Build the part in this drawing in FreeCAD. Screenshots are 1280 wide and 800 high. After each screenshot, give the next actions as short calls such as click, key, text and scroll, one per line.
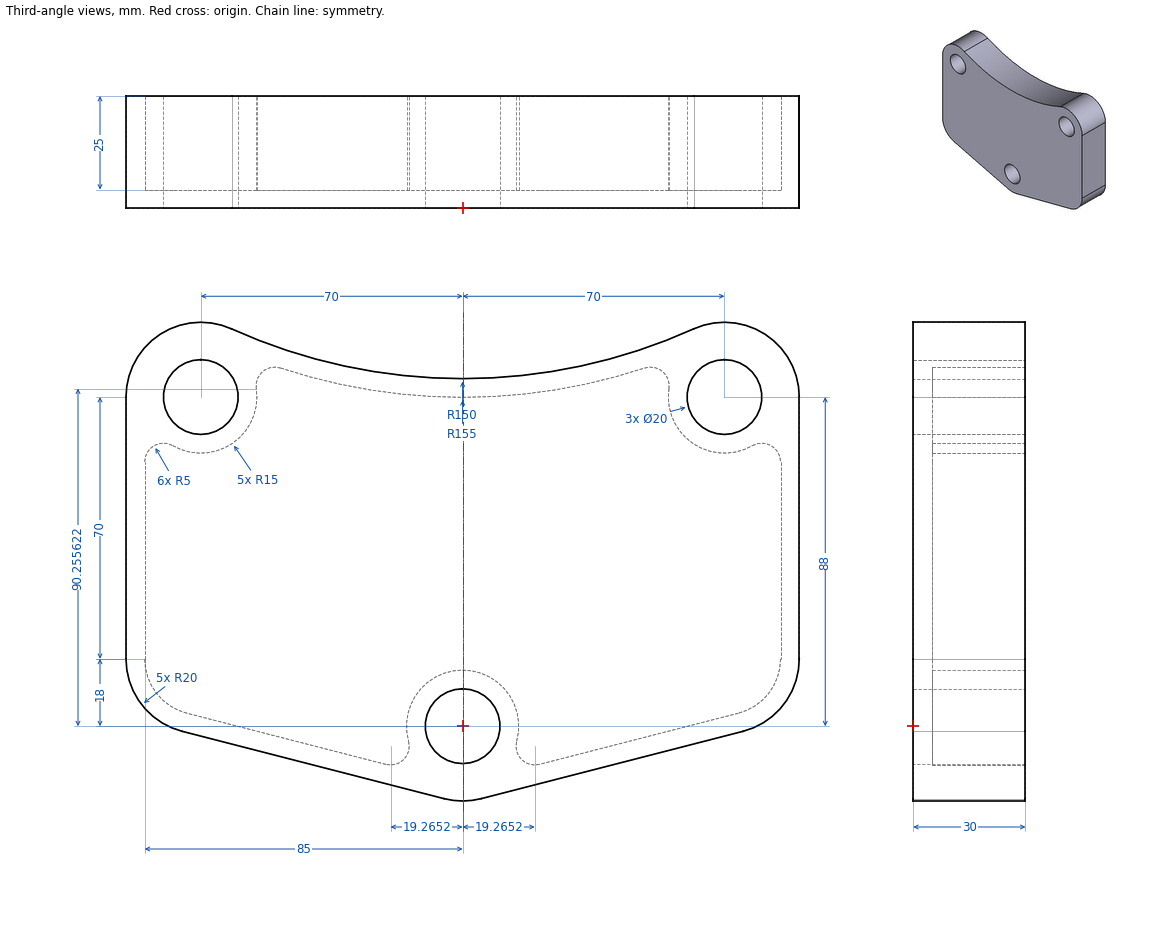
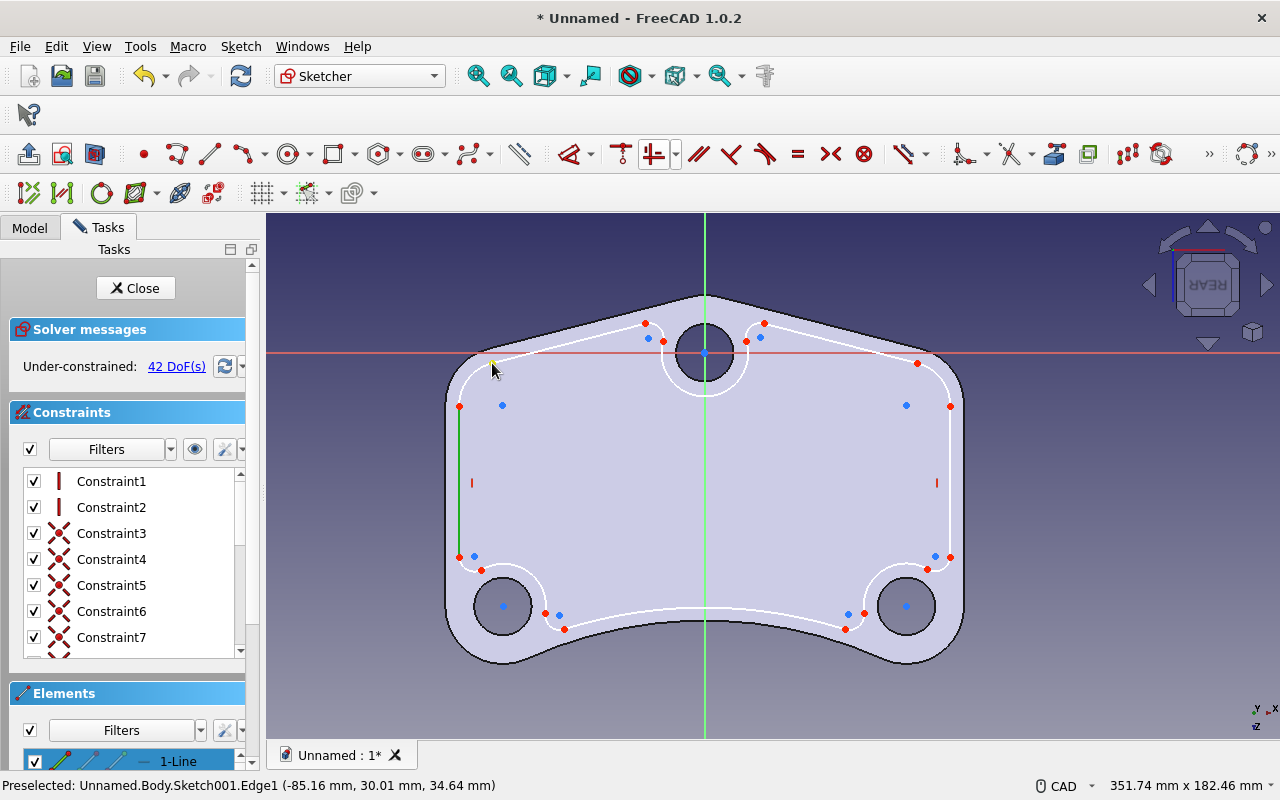
scroll(463, 566, up, 3)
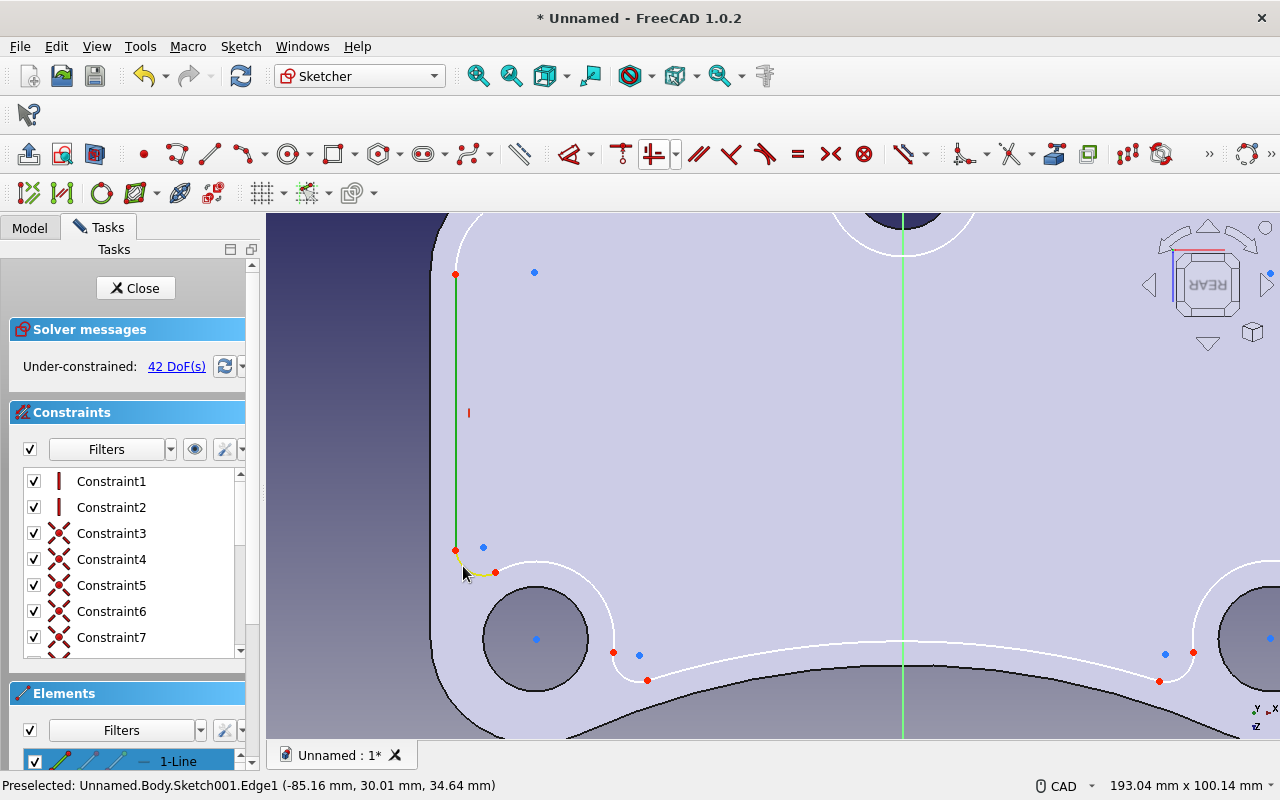
click(462, 565)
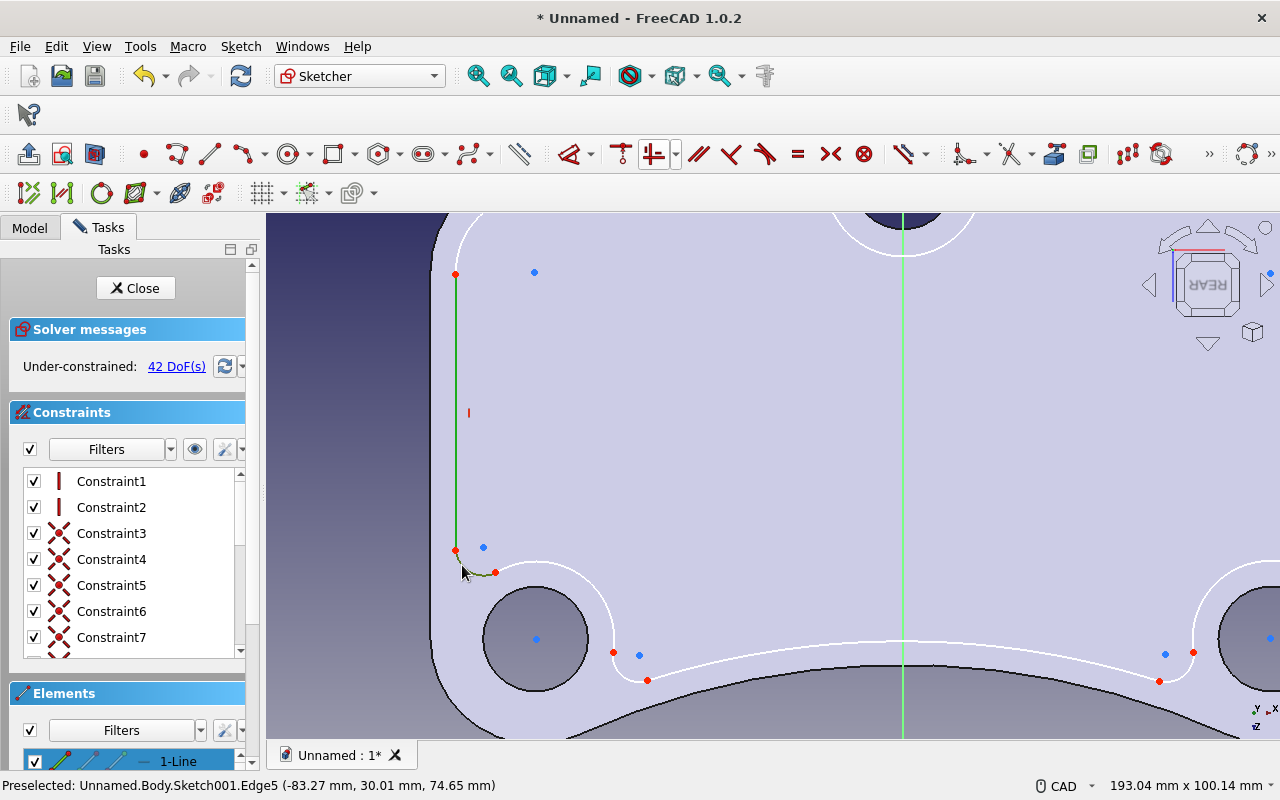
click(765, 154)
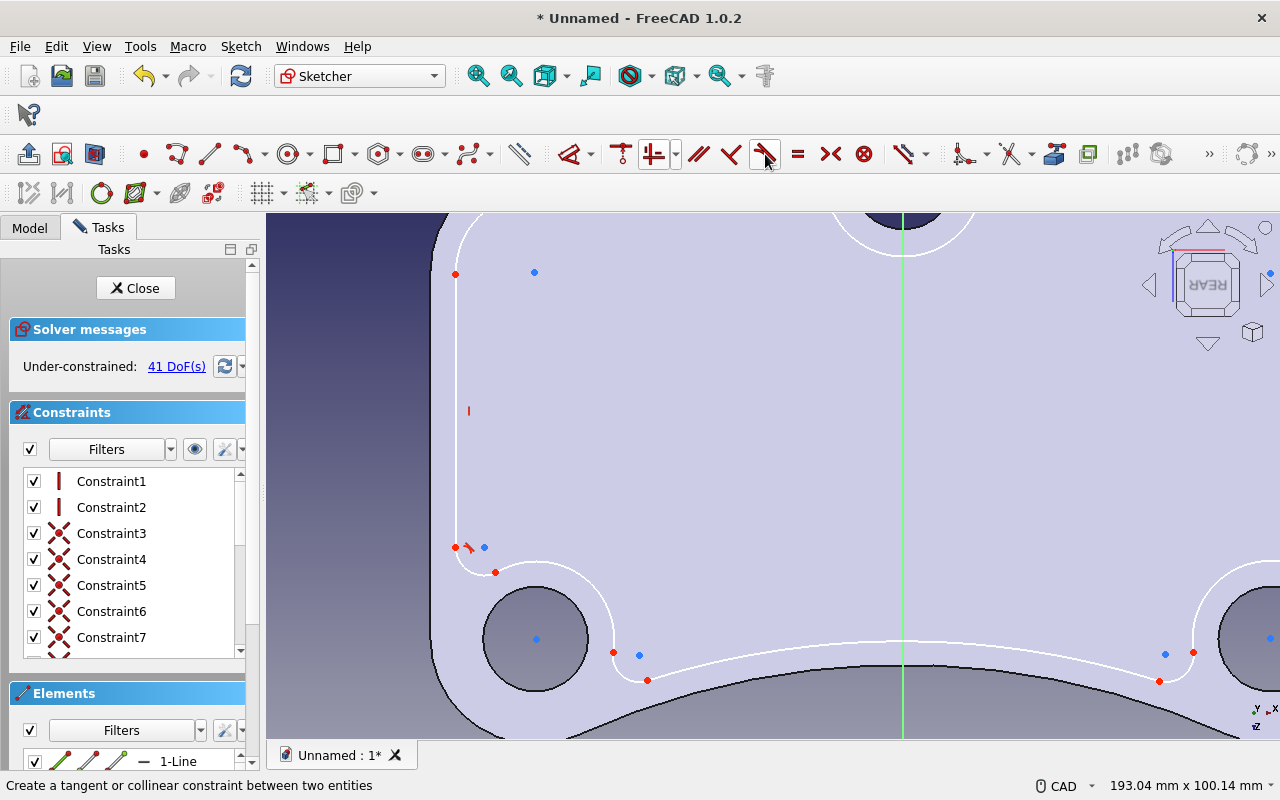
click(456, 356)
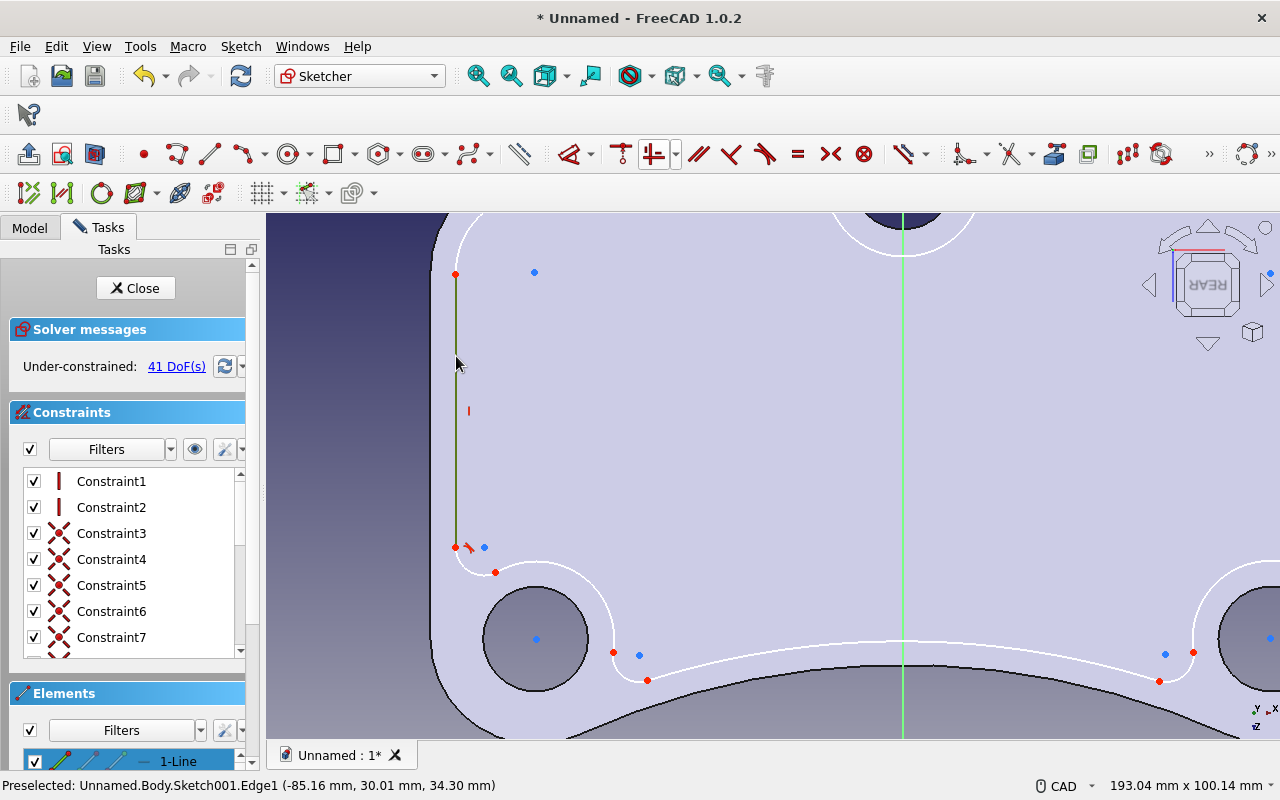
click(462, 243)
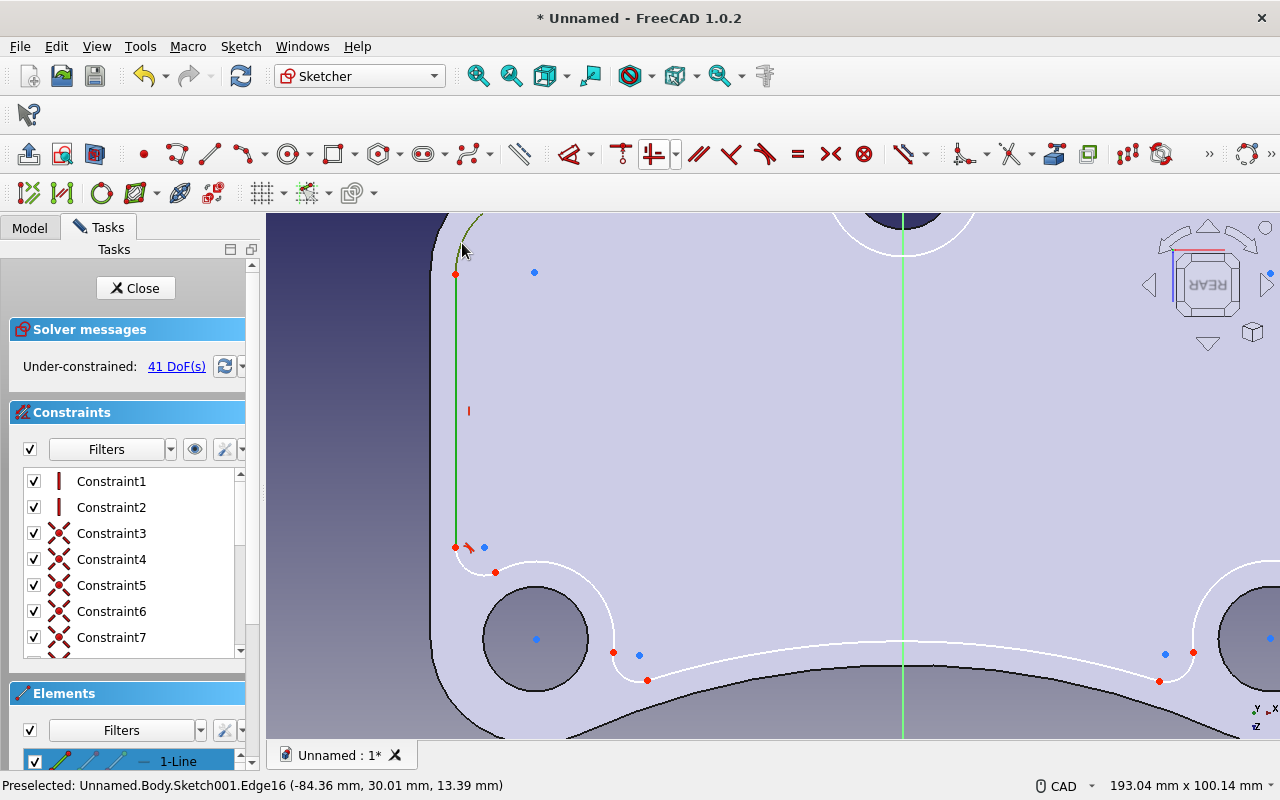
click(765, 154)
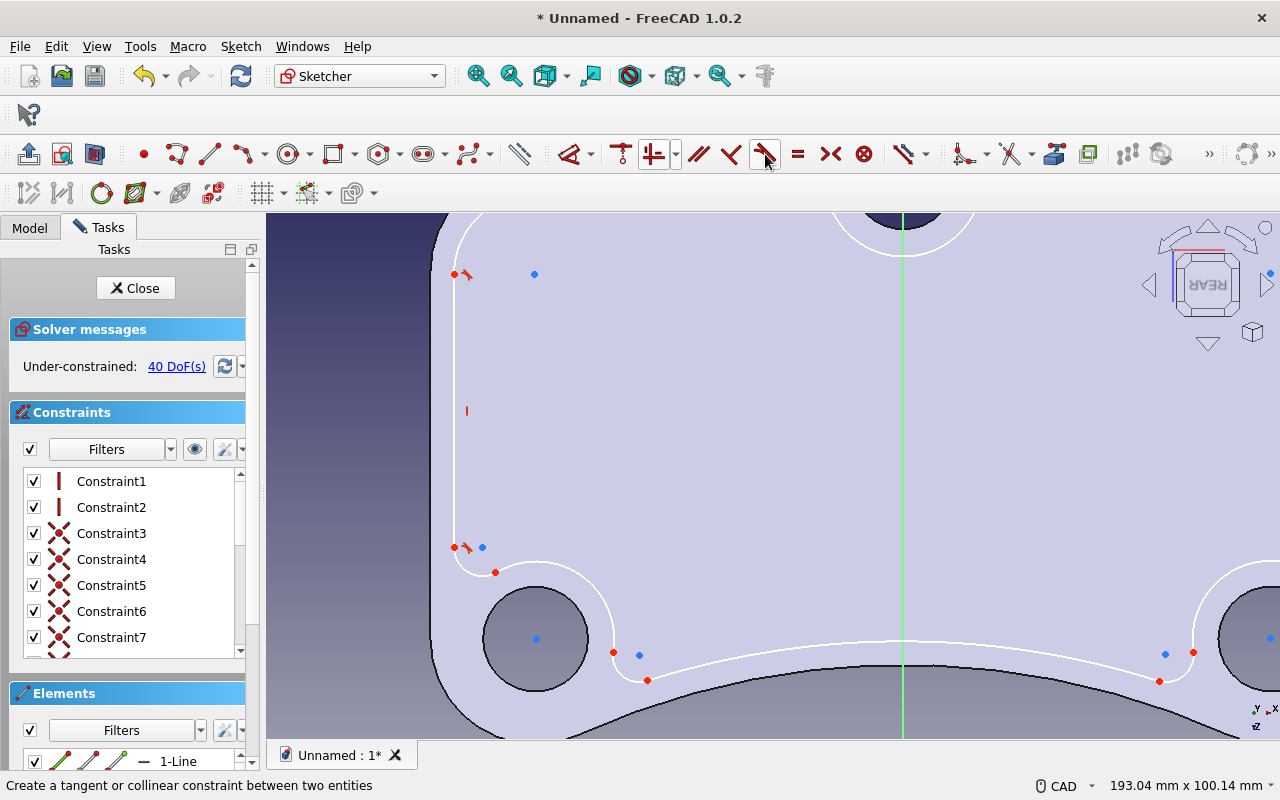
scroll(463, 567, down, 3)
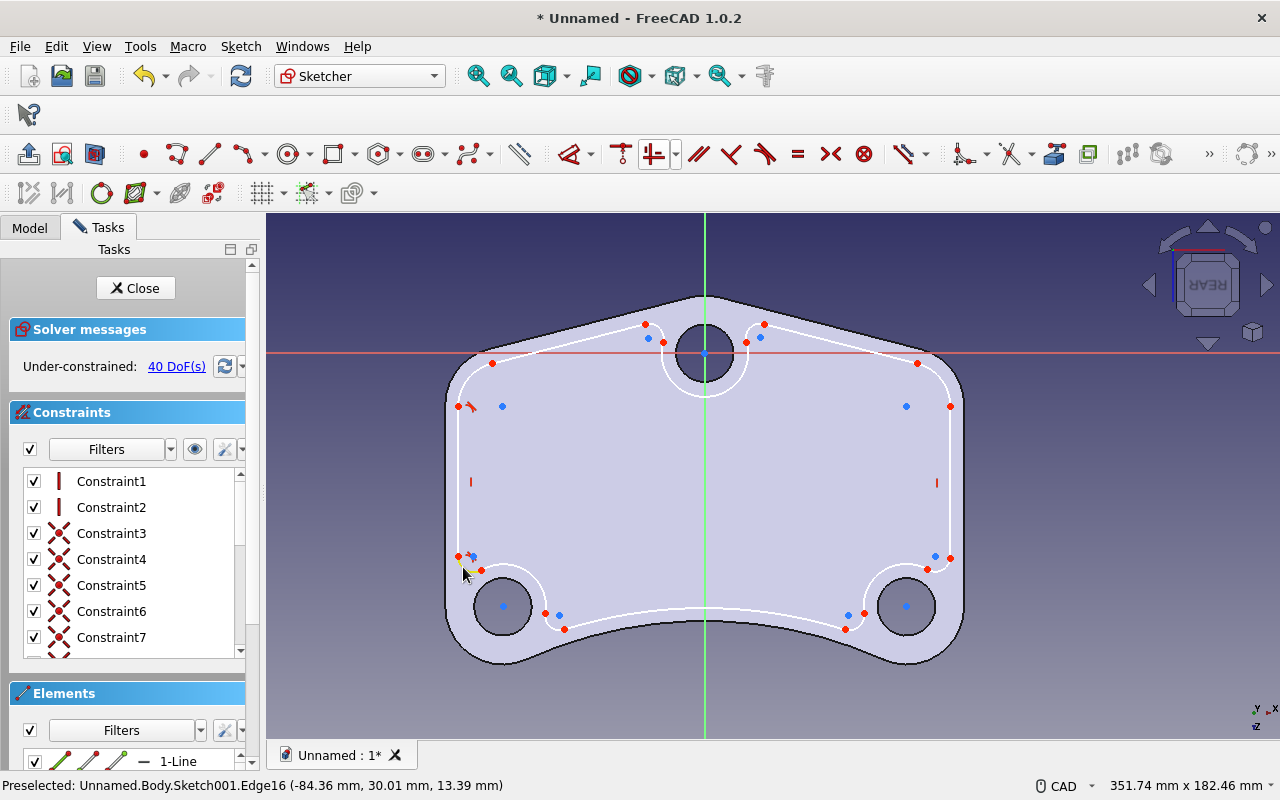
click(950, 513)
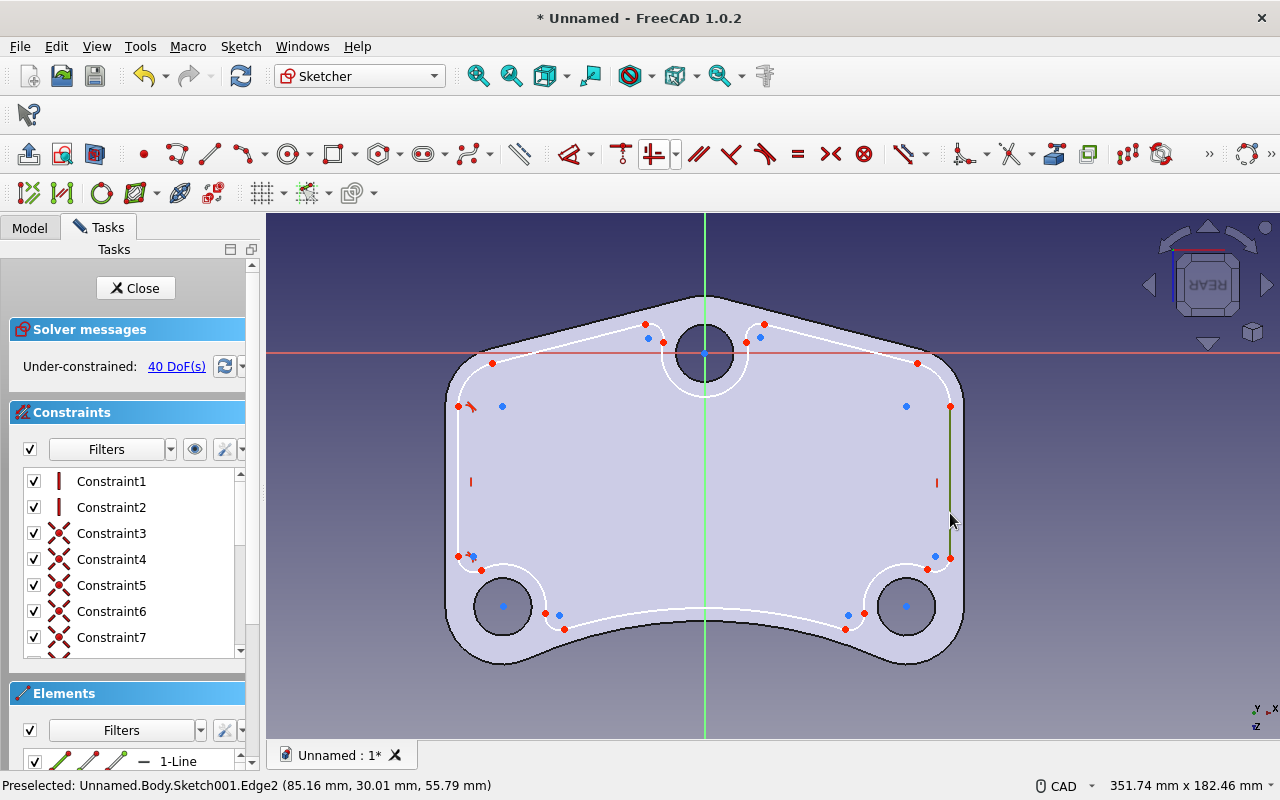
click(942, 570)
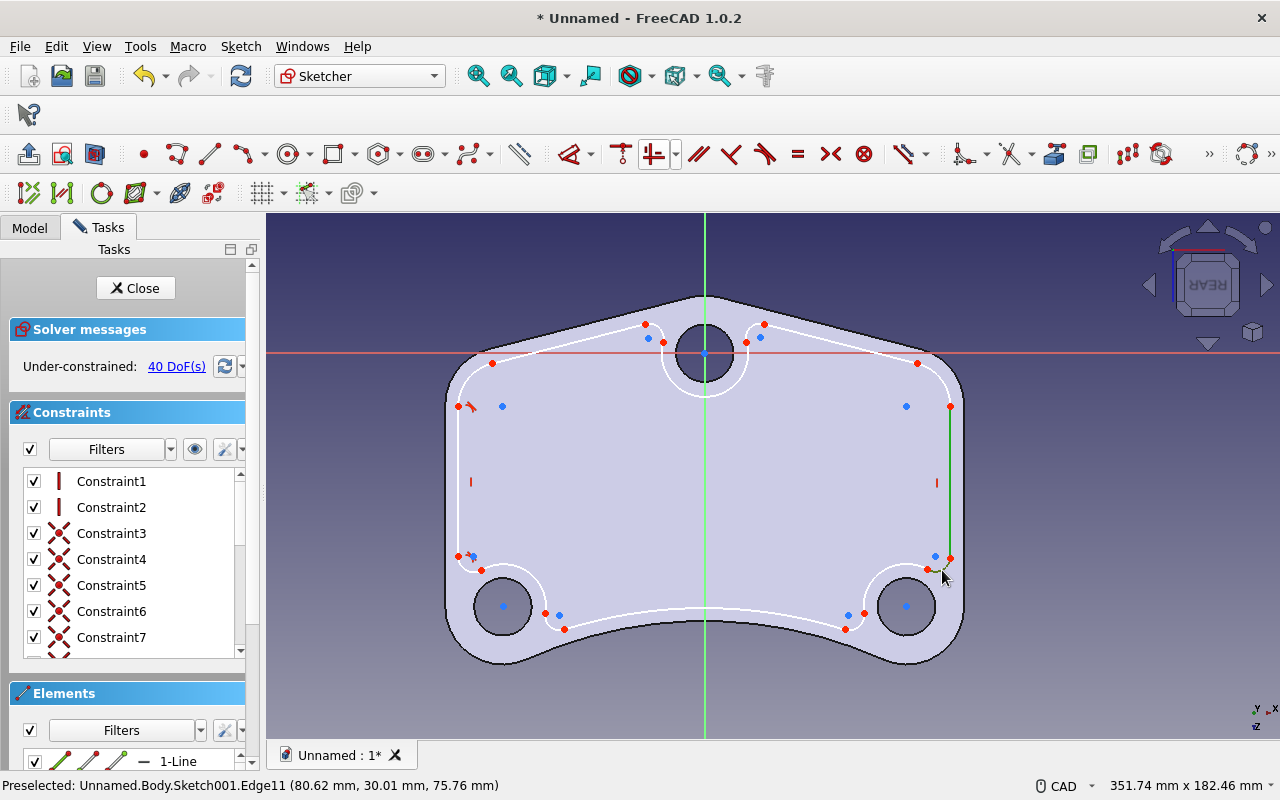
click(765, 154)